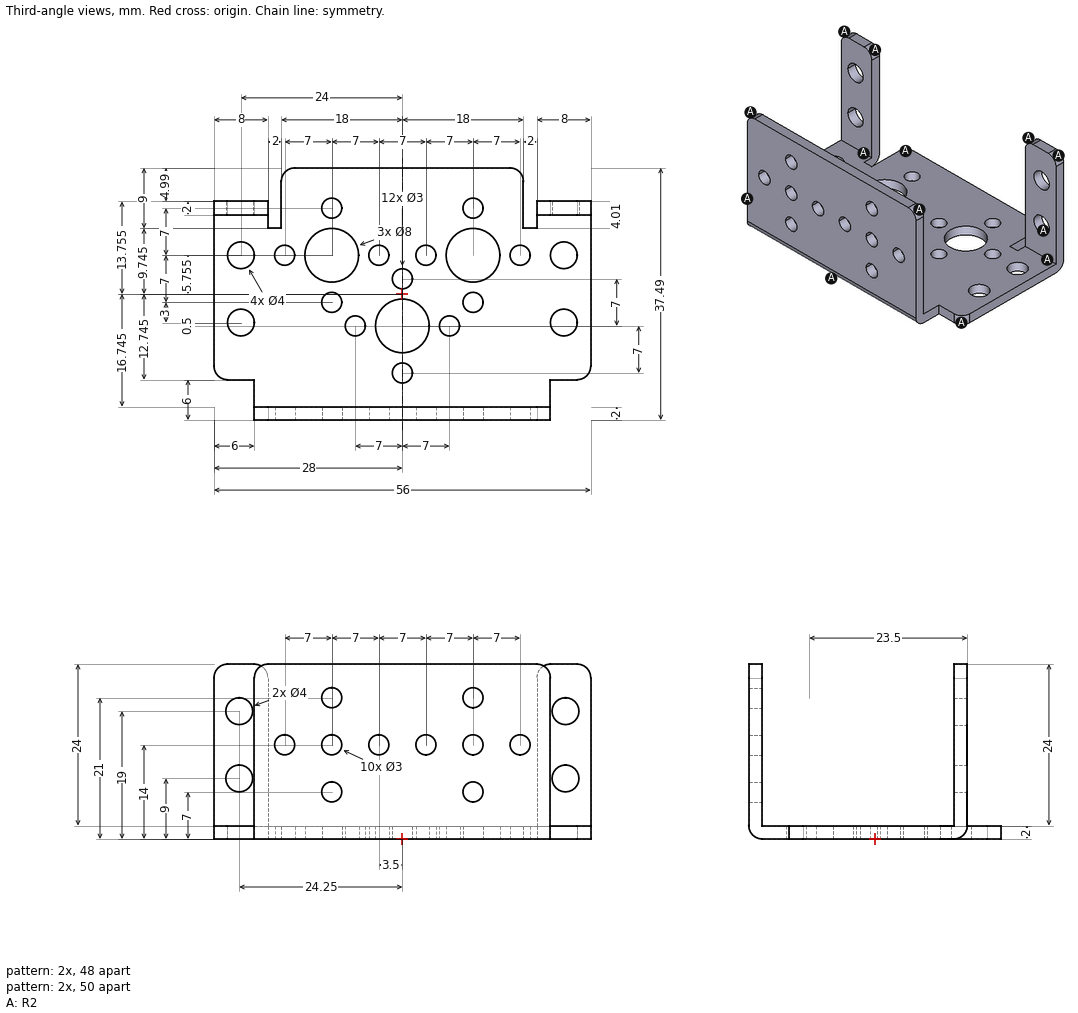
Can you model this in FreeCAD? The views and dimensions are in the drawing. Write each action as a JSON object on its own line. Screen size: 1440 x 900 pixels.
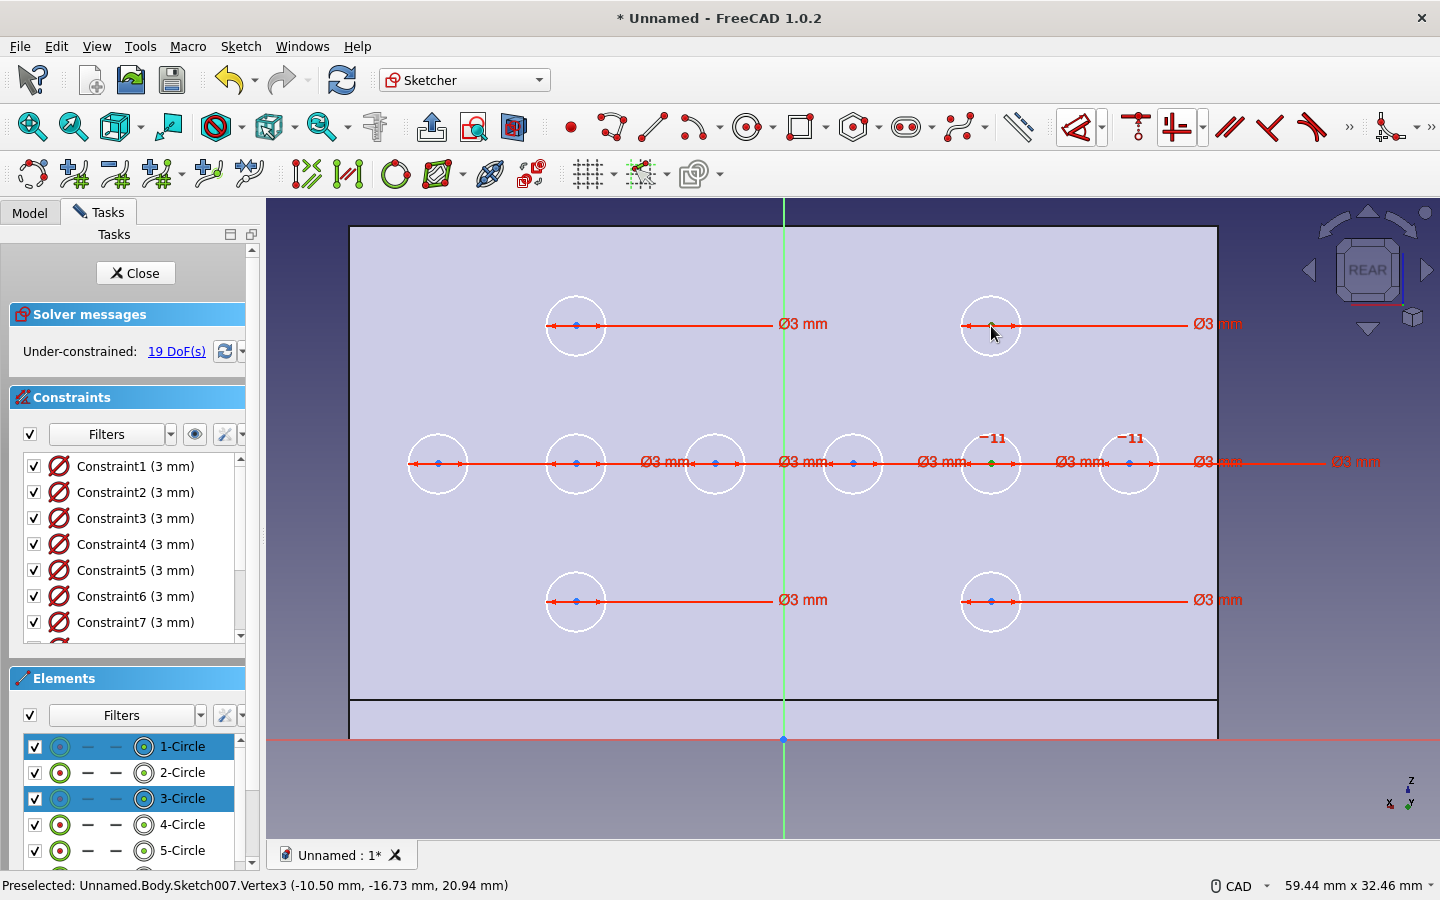
{"action": "key", "text": "v"}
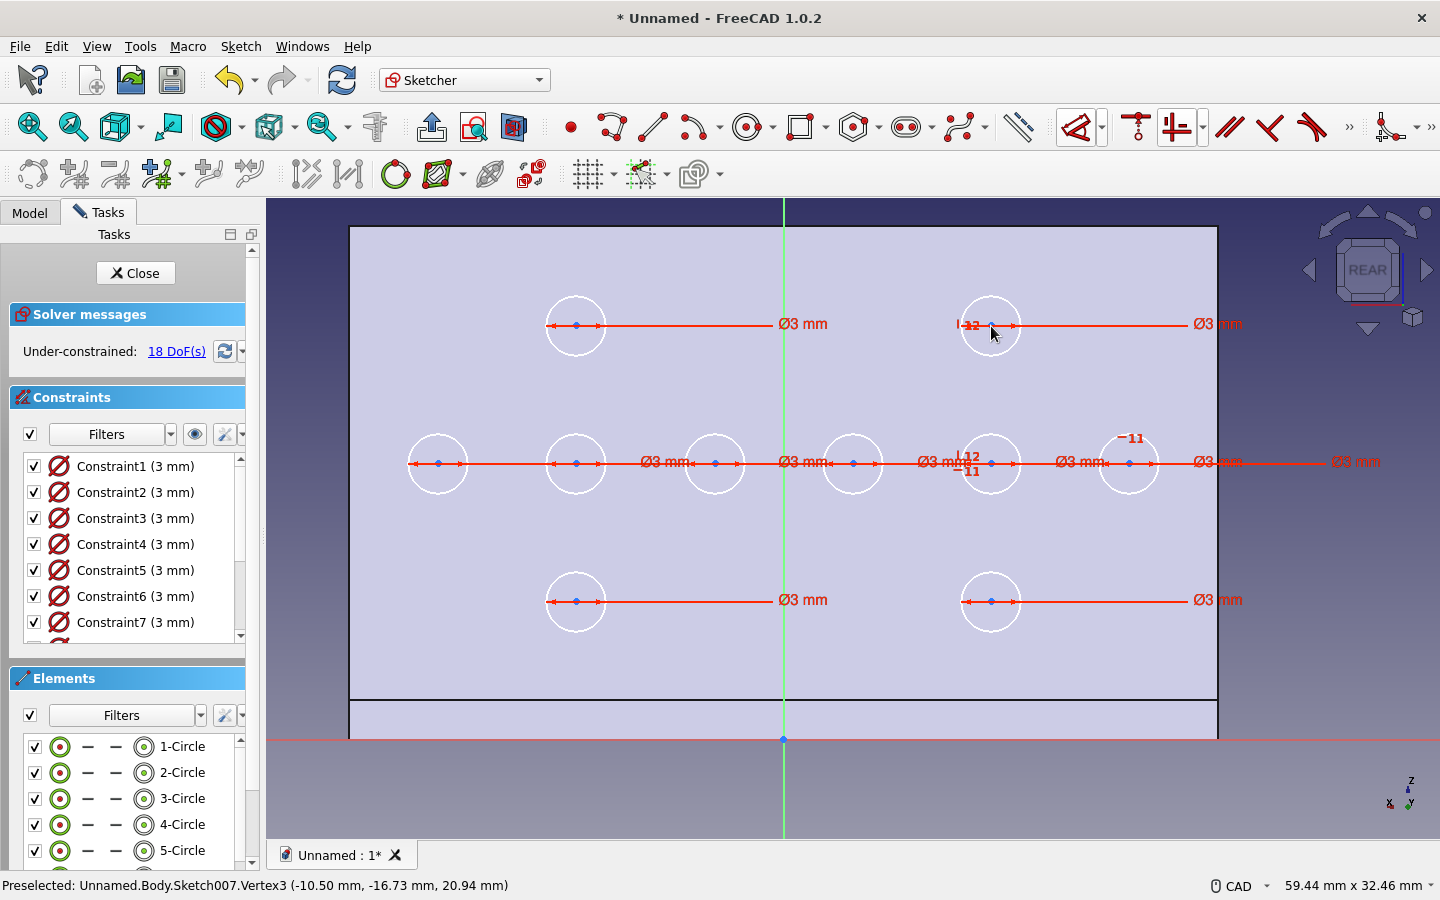
{"action": "left_click", "coordinate": [991, 464]}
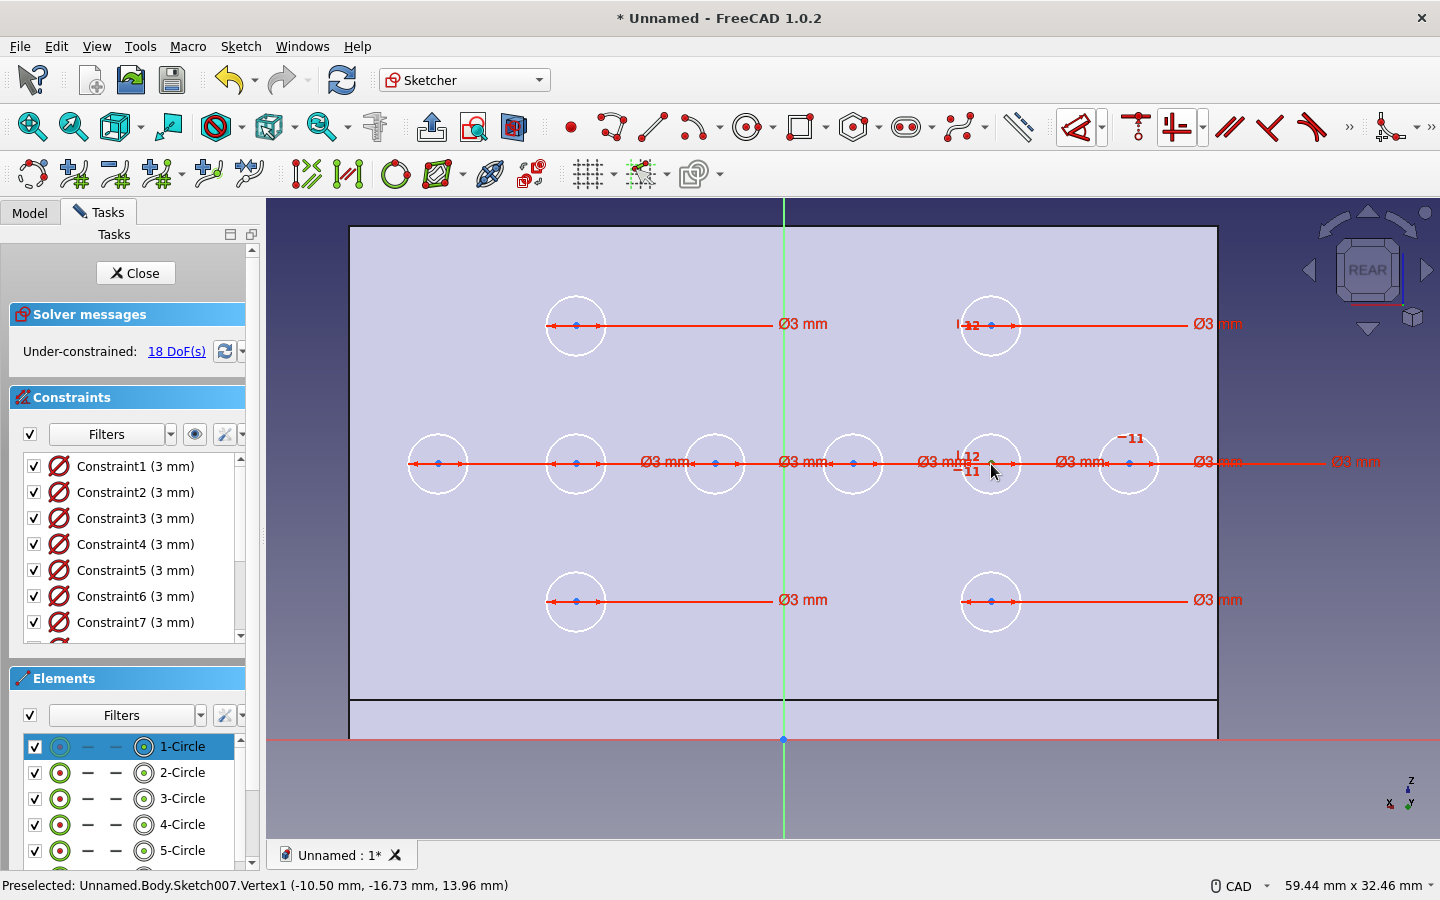
{"action": "left_click", "coordinate": [853, 464]}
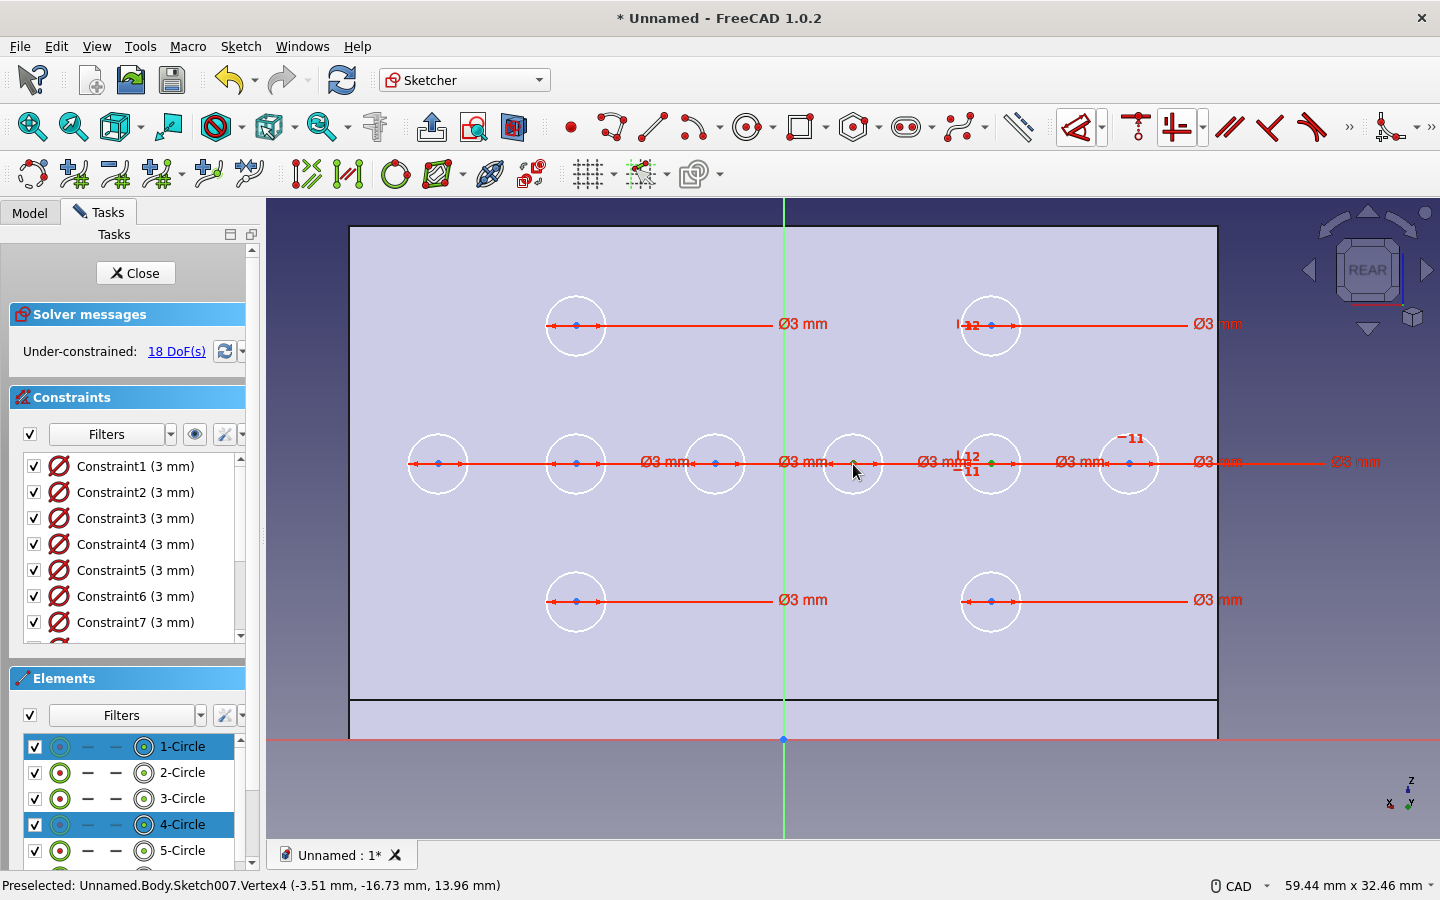
{"action": "key", "text": "h"}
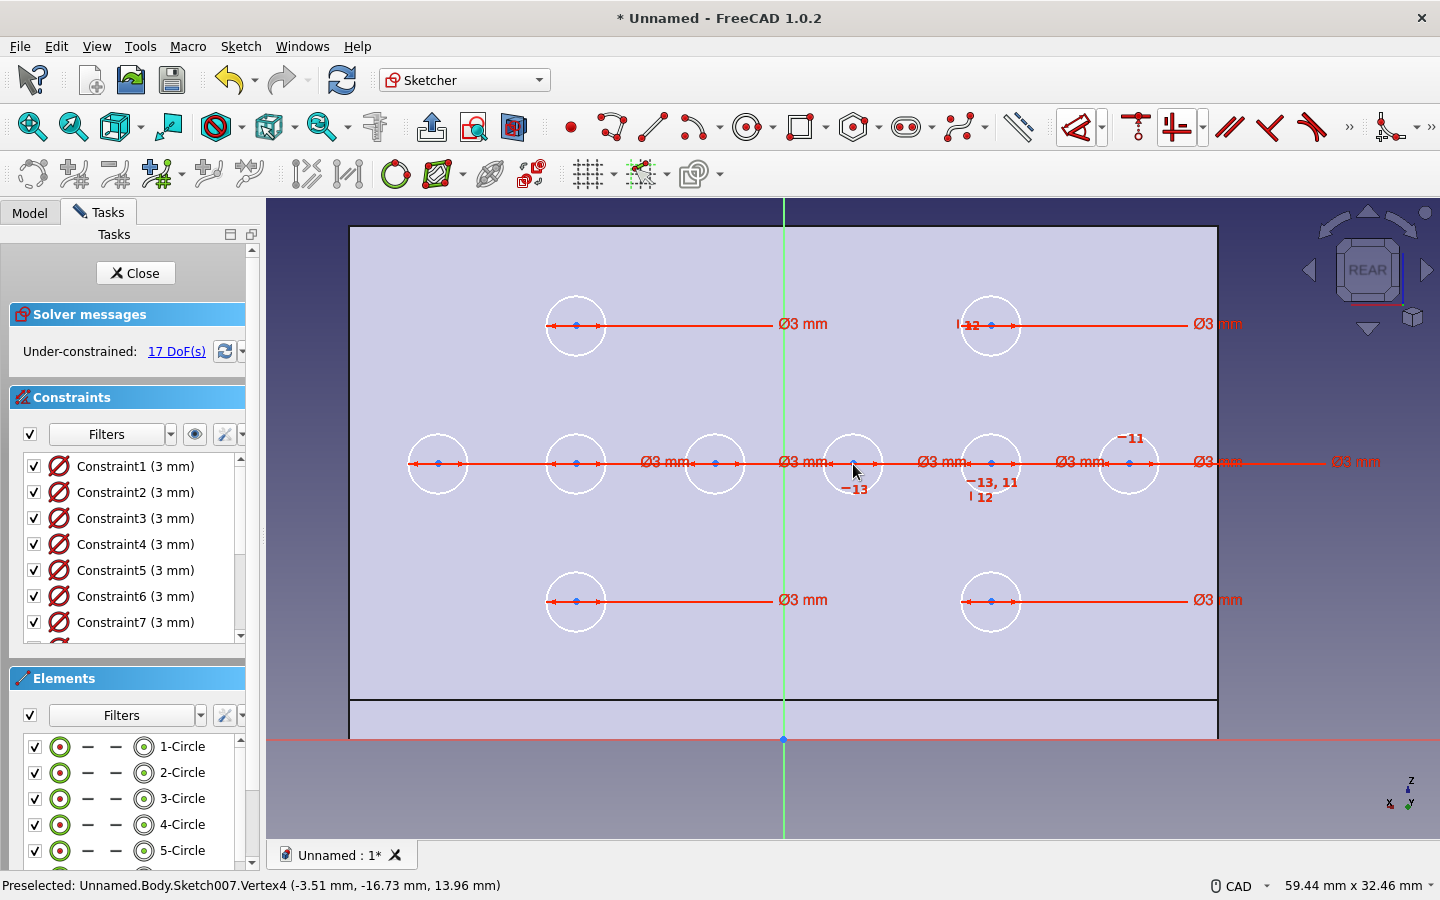
{"action": "left_click", "coordinate": [991, 464]}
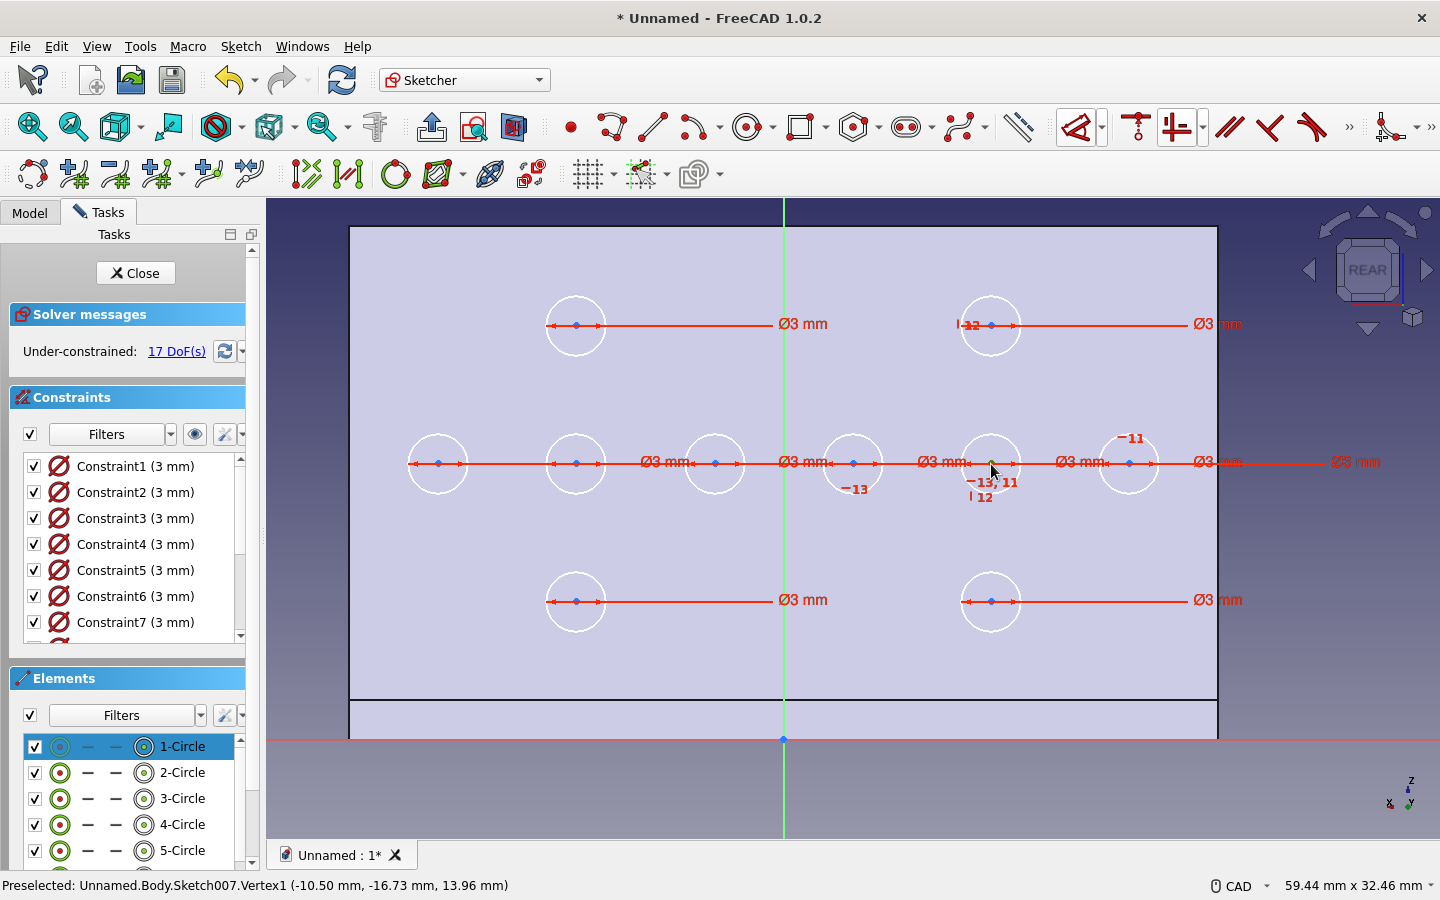
{"action": "left_click", "coordinate": [991, 602]}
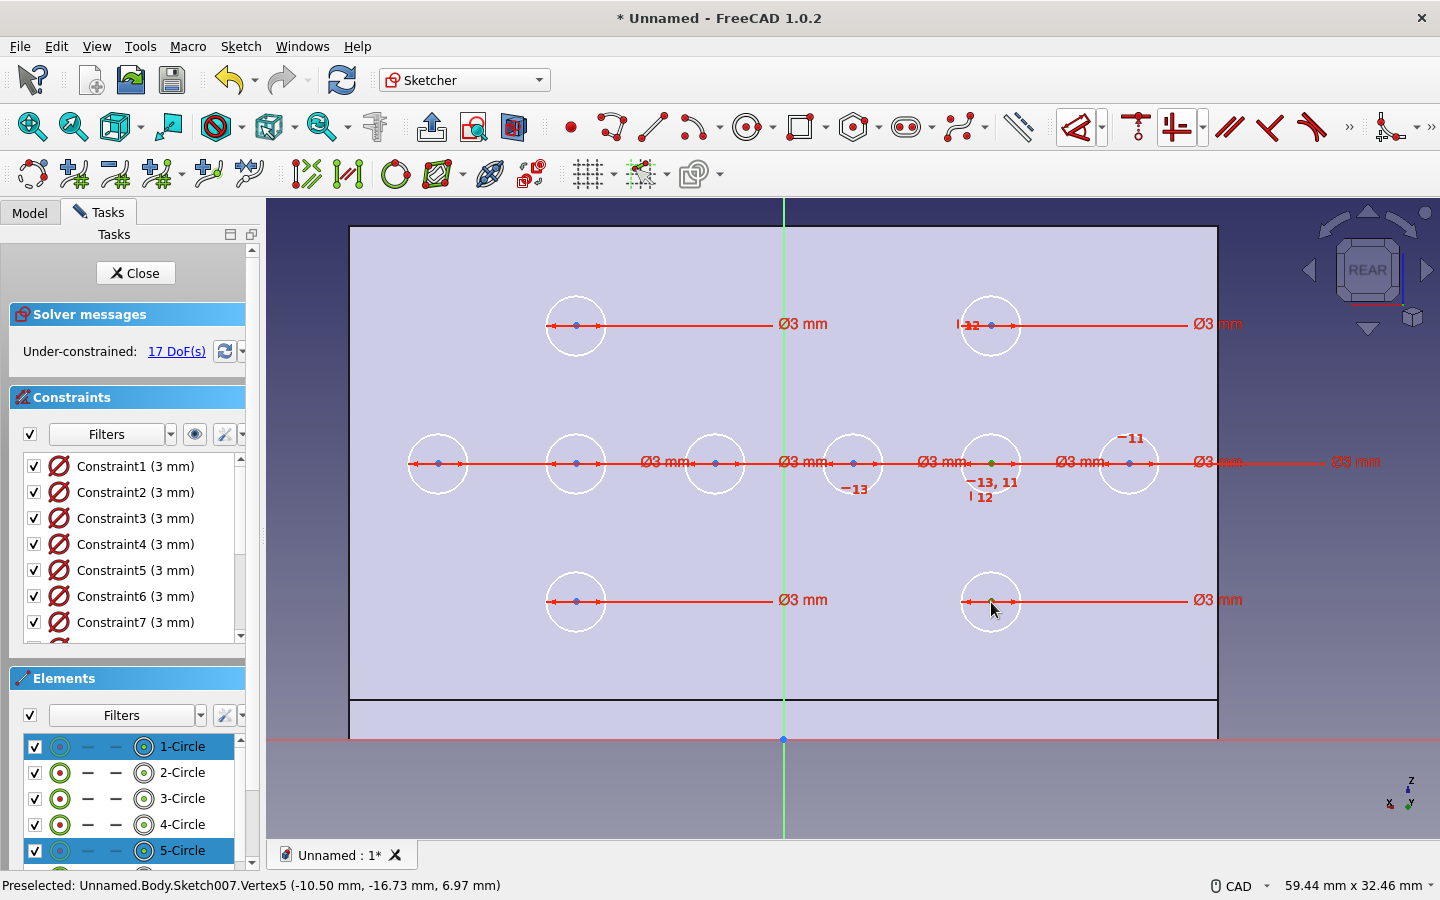
{"action": "key", "text": "v"}